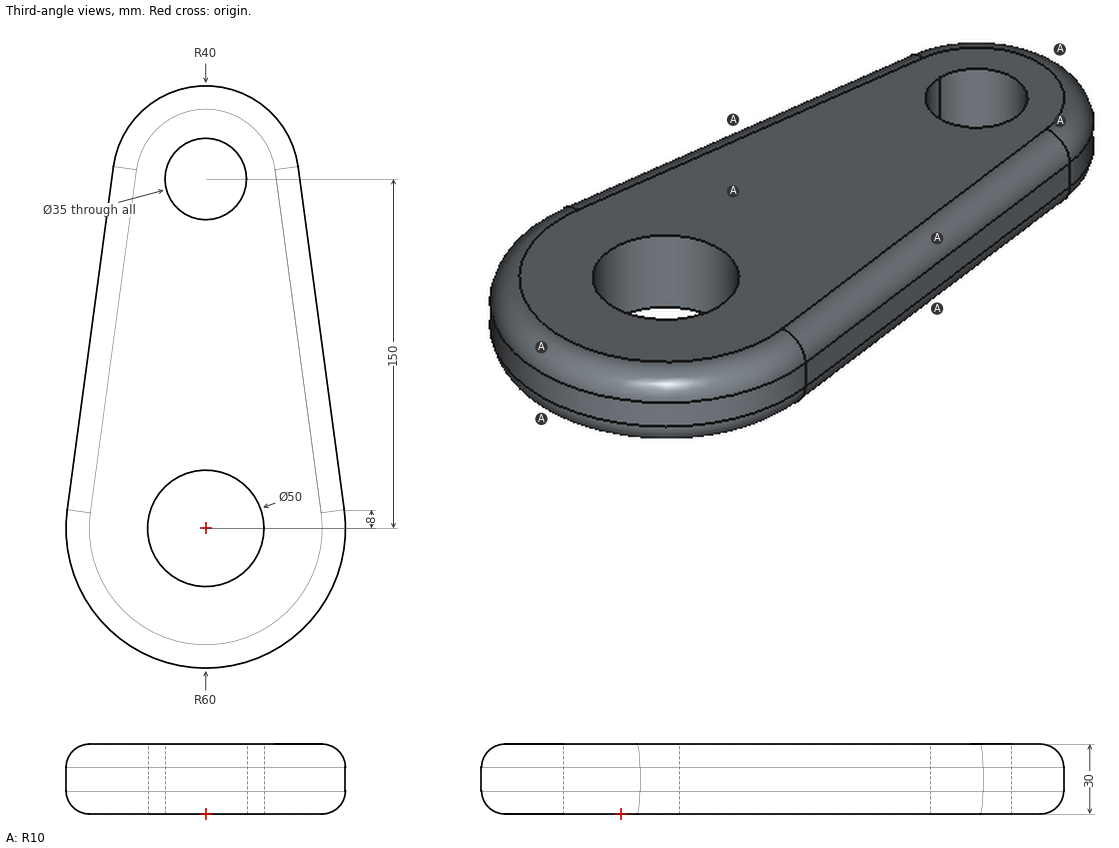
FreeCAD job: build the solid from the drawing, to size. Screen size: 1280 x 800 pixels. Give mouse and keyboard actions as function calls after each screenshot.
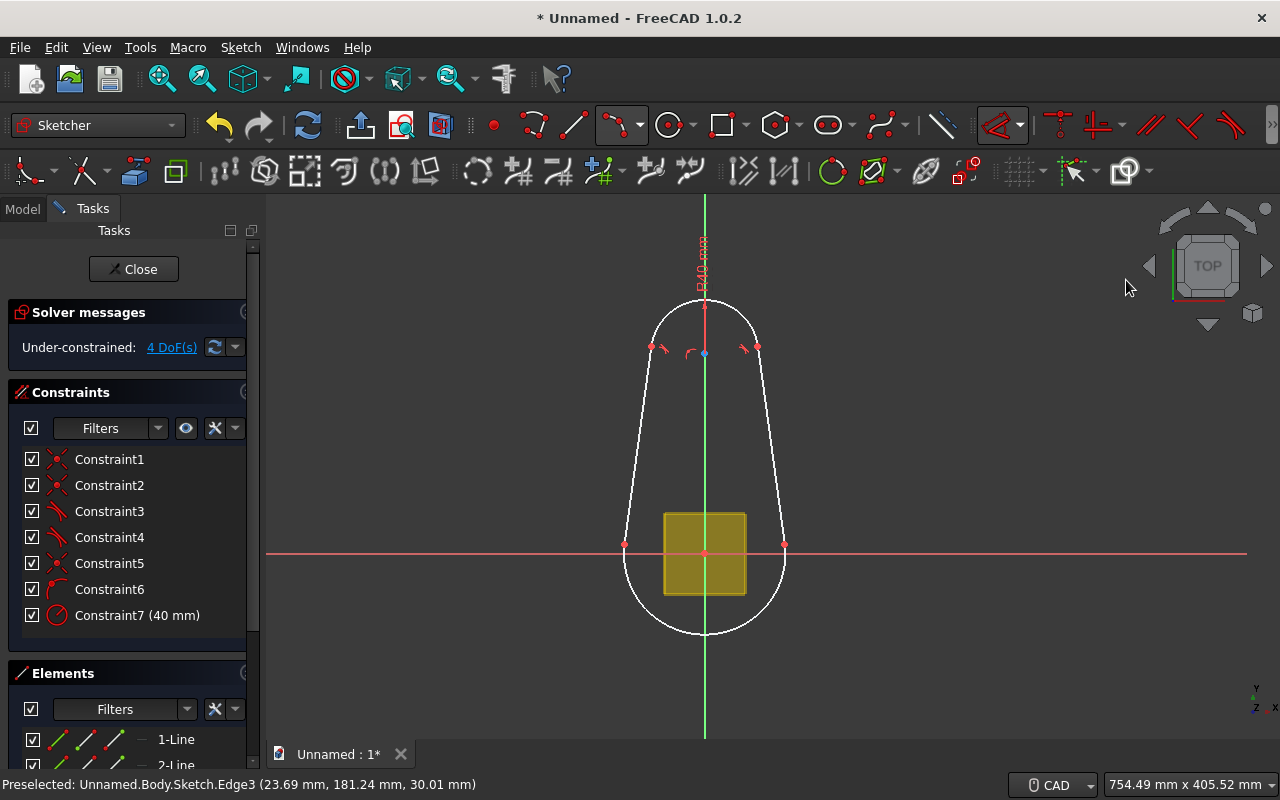
click(654, 617)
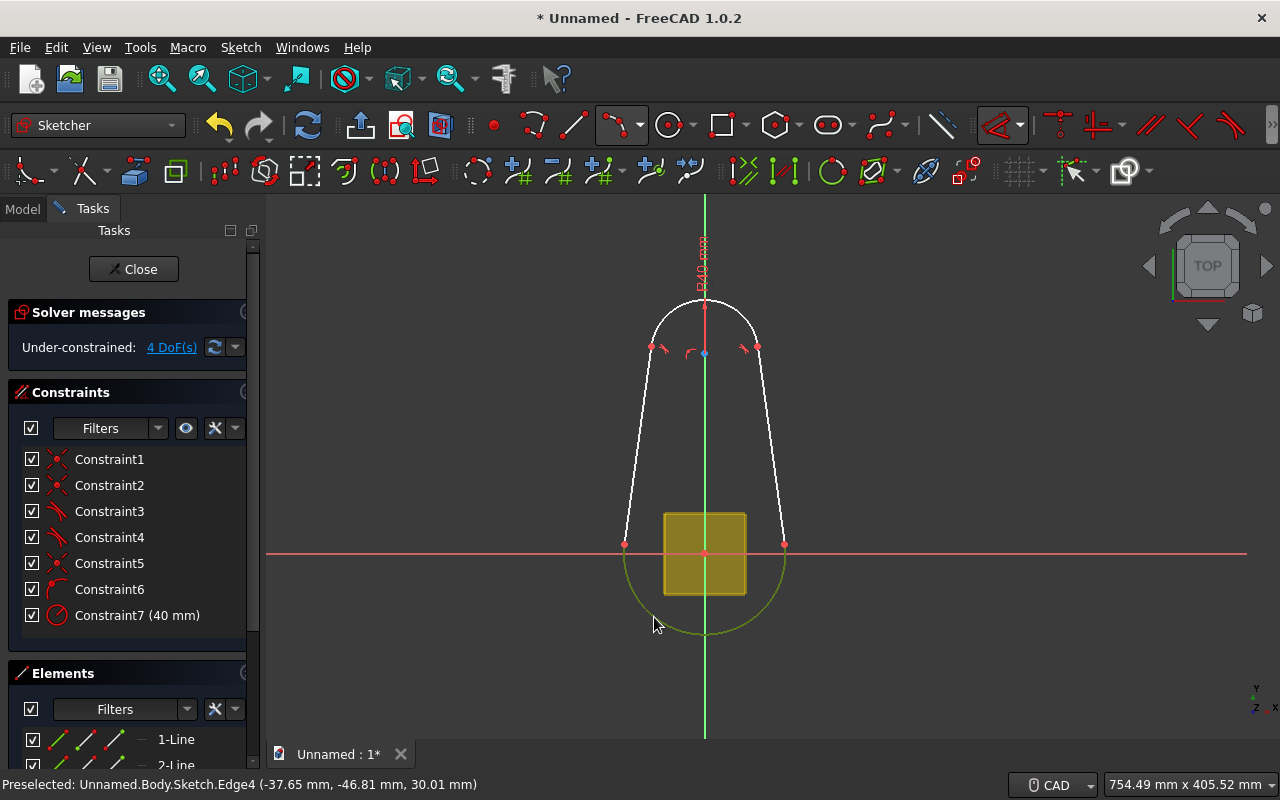
key(k)
key(r)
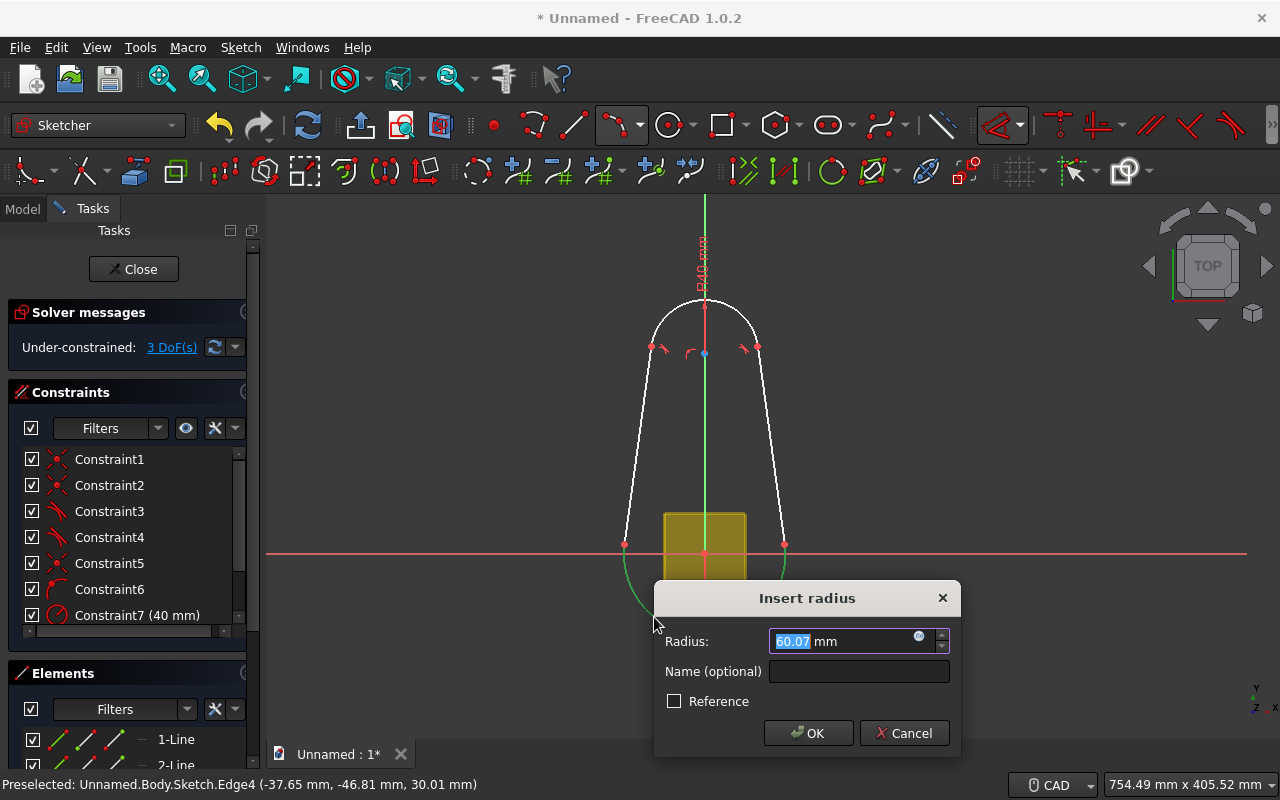
text(60)
key(Return)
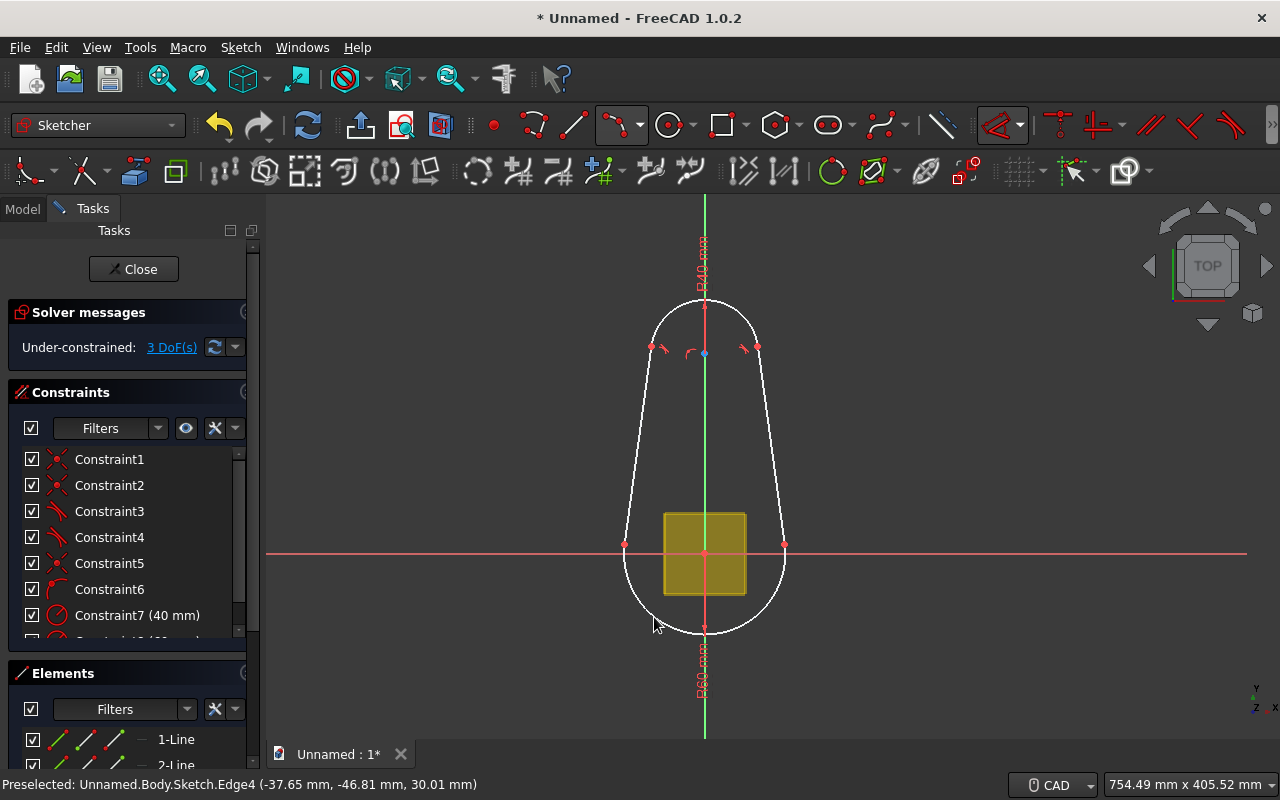
scroll(785, 544, up, 7)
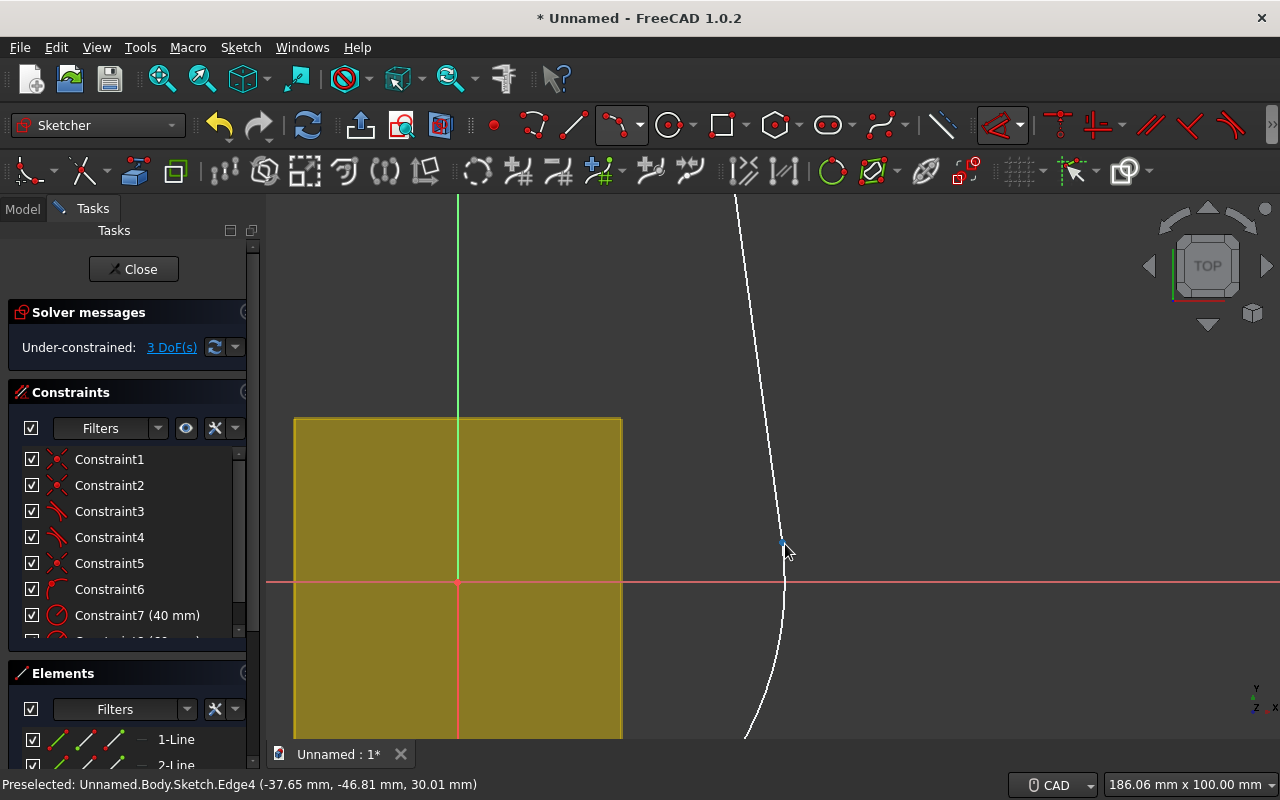
click(782, 542)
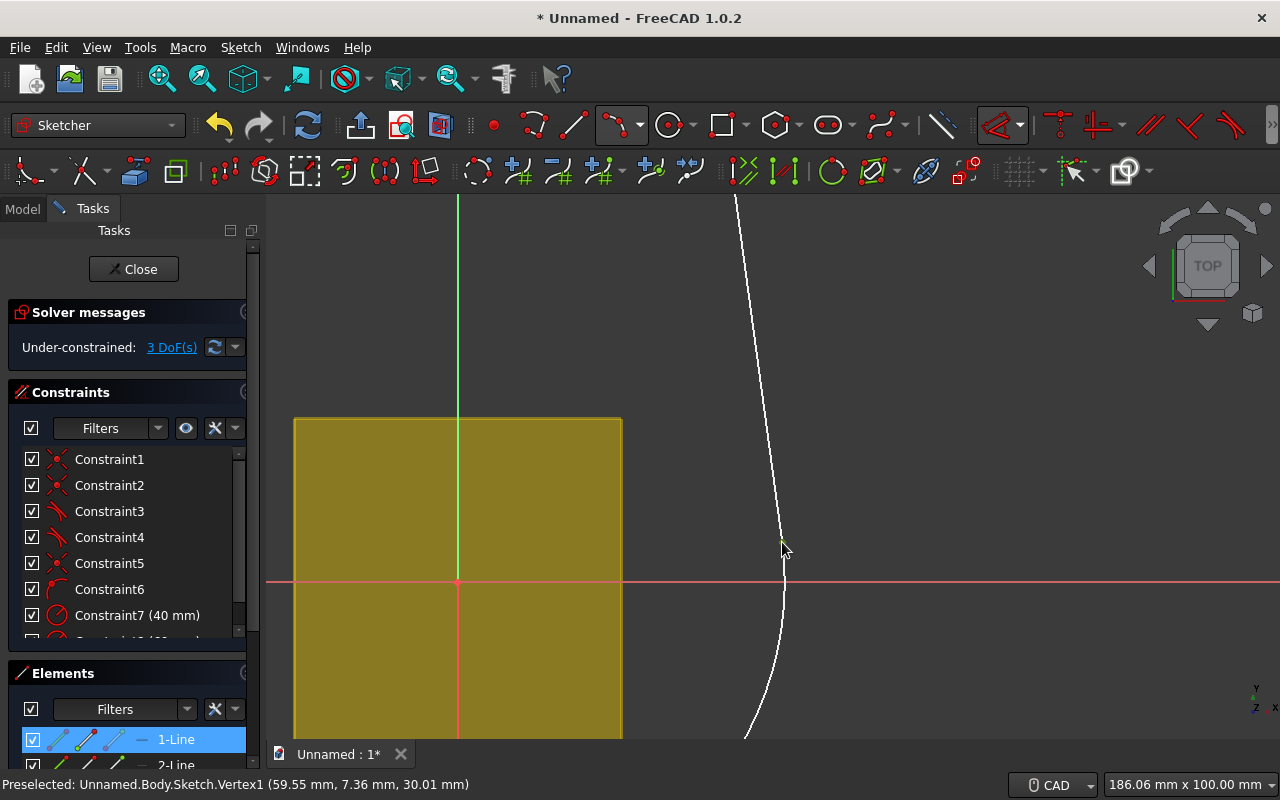
click(1022, 126)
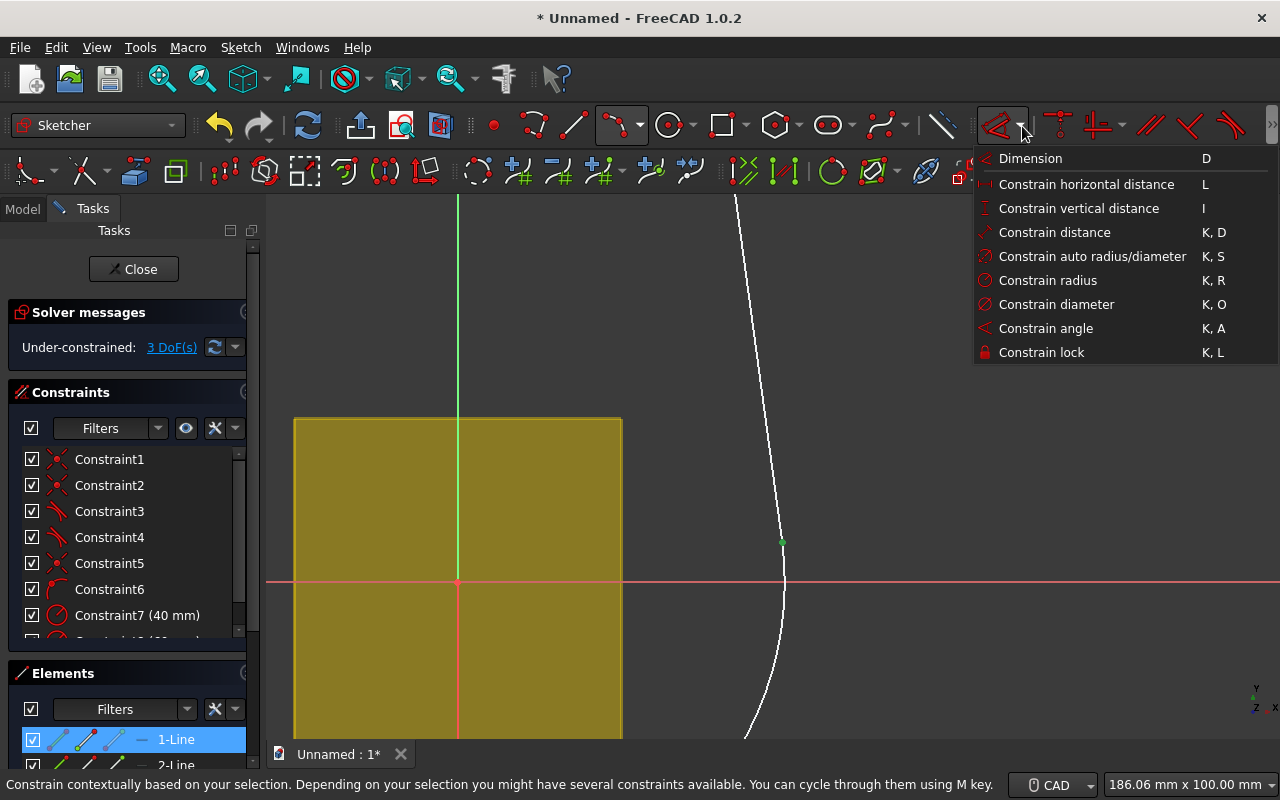
click(1126, 208)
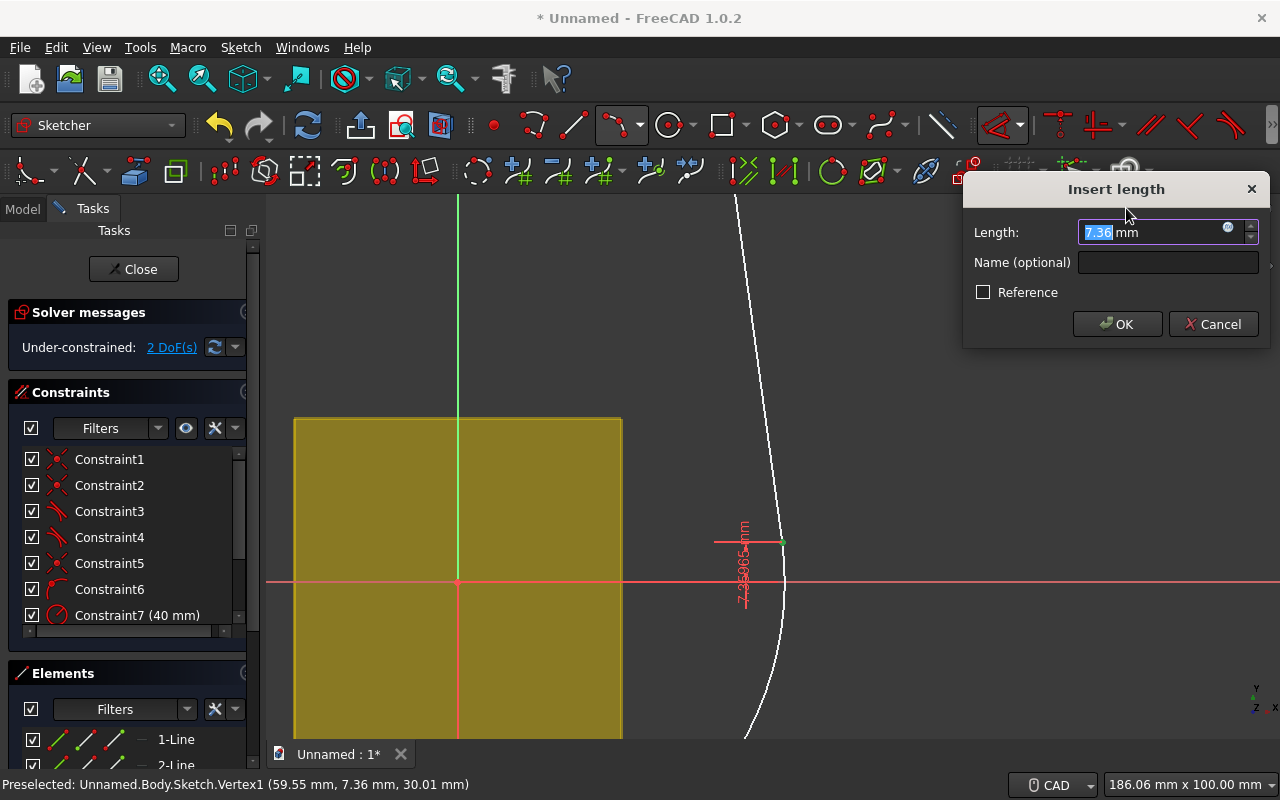
text(8)
key(Return)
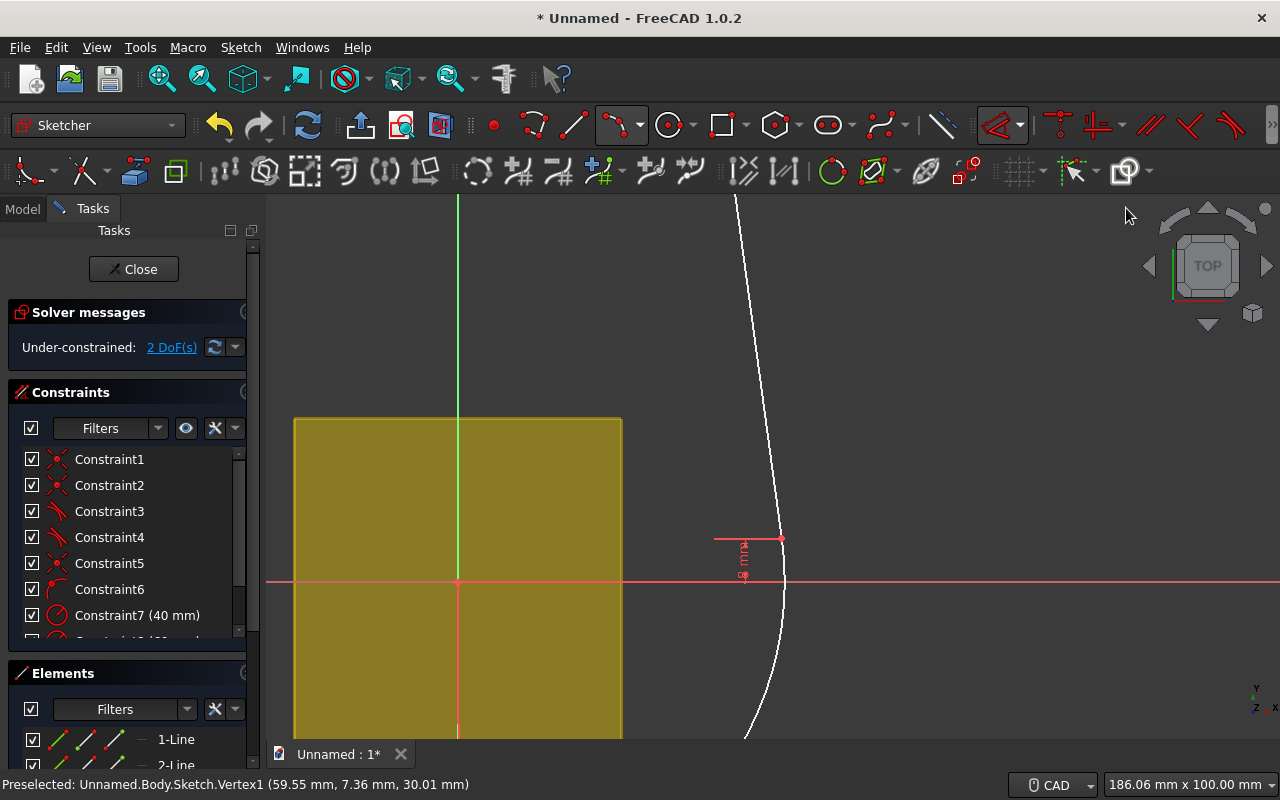
scroll(785, 545, down, 7)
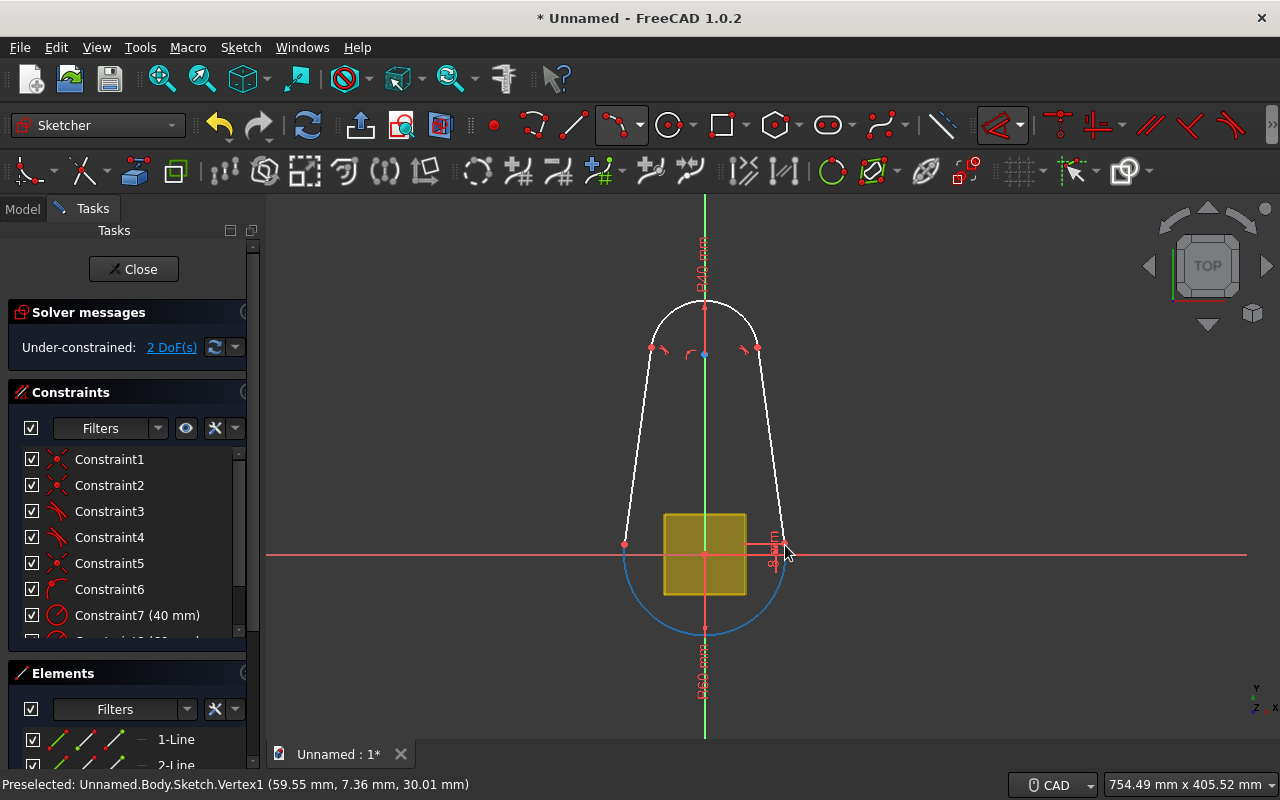
scroll(625, 545, up, 7)